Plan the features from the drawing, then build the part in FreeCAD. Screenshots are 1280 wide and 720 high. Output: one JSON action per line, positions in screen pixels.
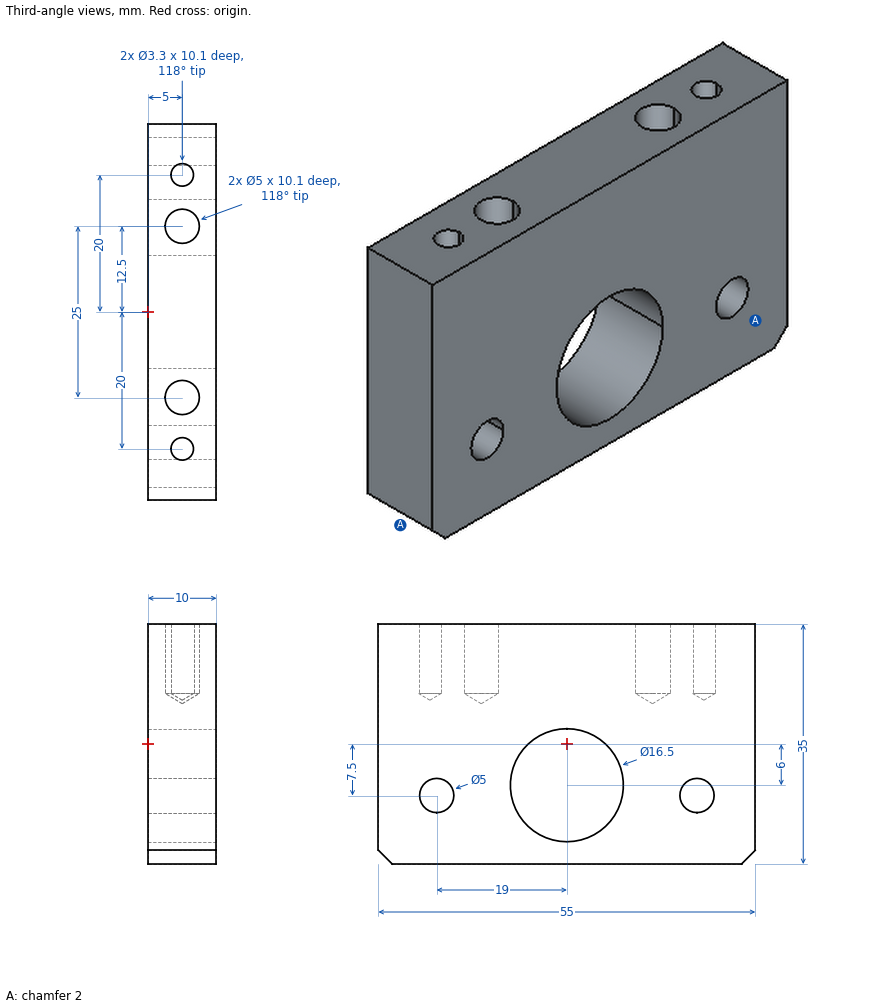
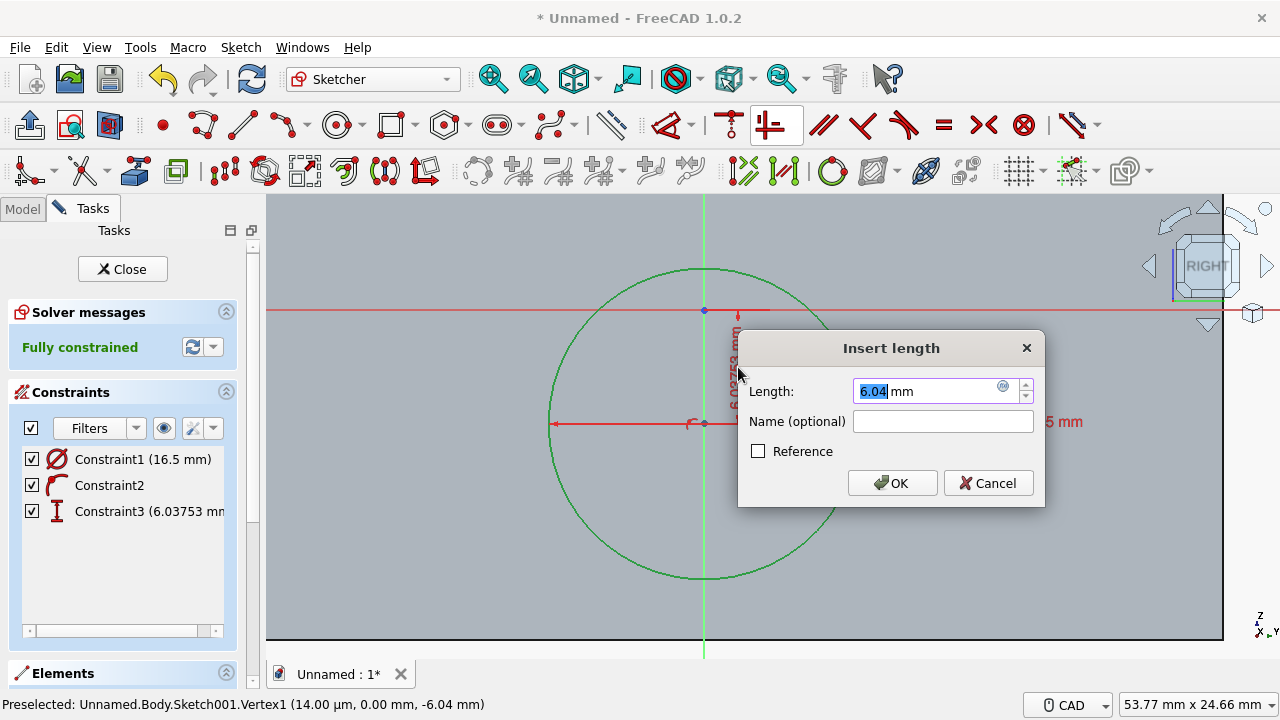
{"action": "type", "text": "6"}
{"action": "key", "text": "Return"}
{"action": "key", "text": "Escape"}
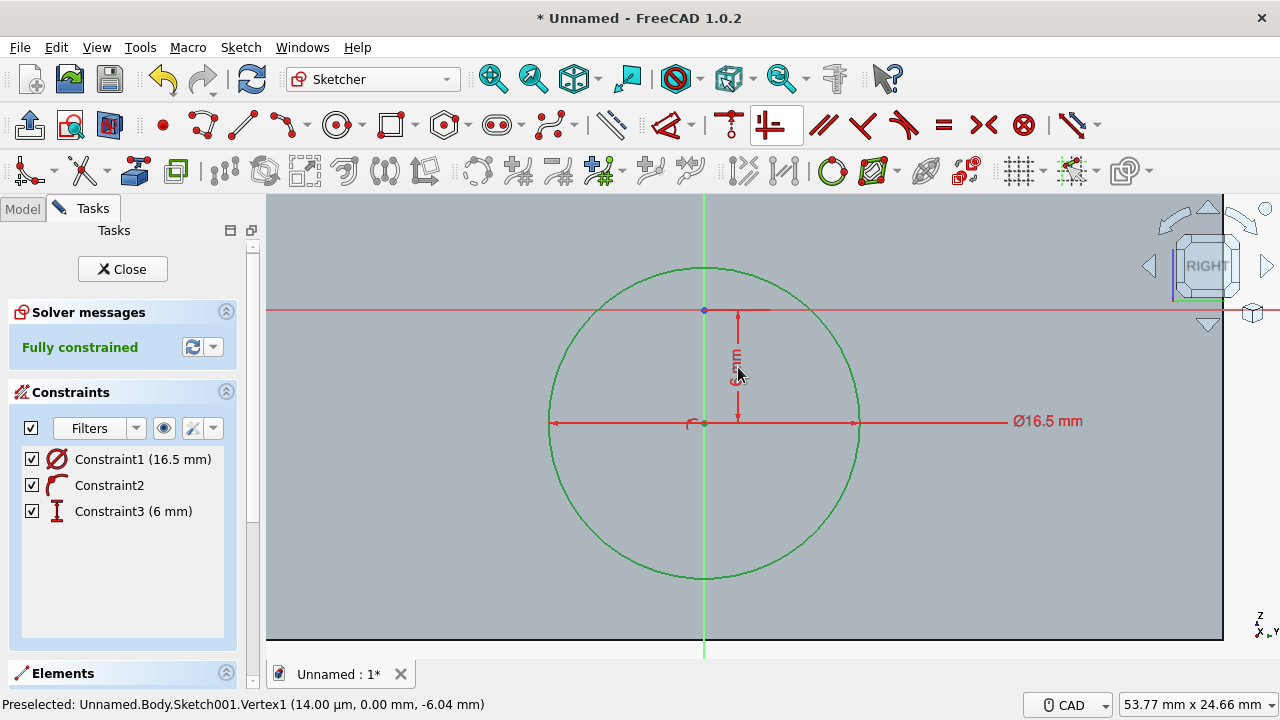
{"action": "left_click", "coordinate": [123, 269]}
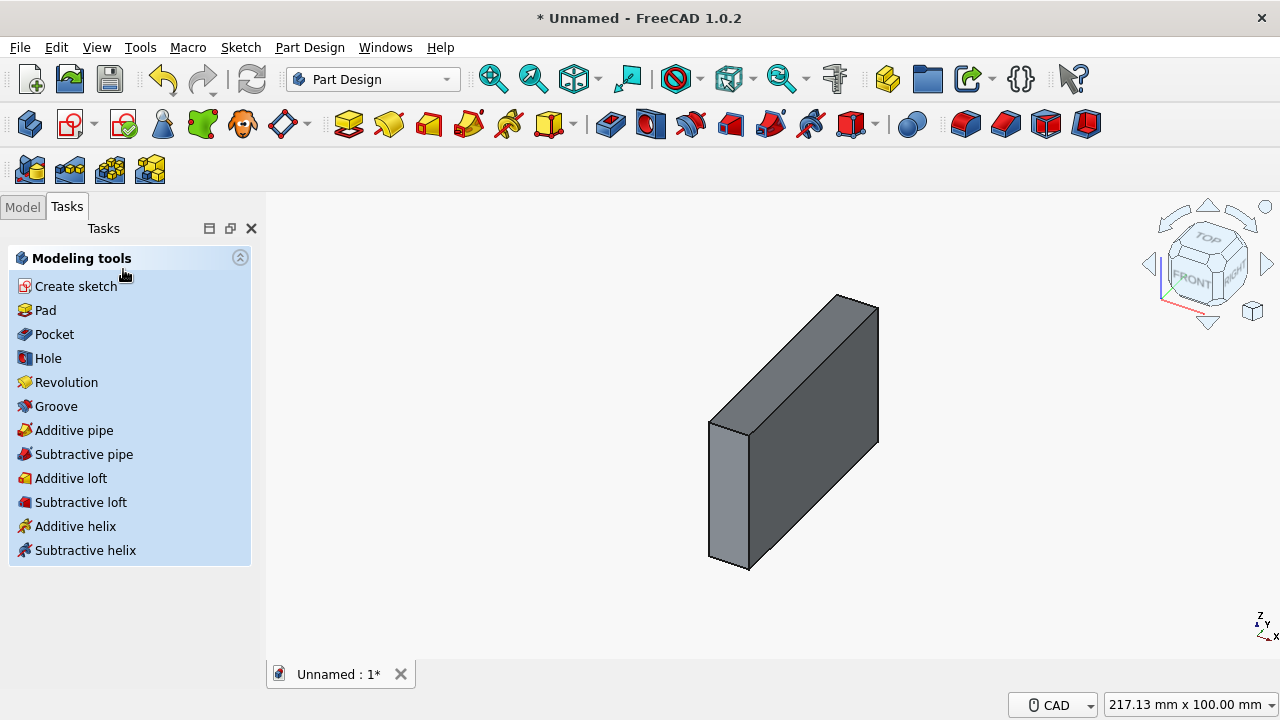
{"action": "left_click", "coordinate": [612, 124]}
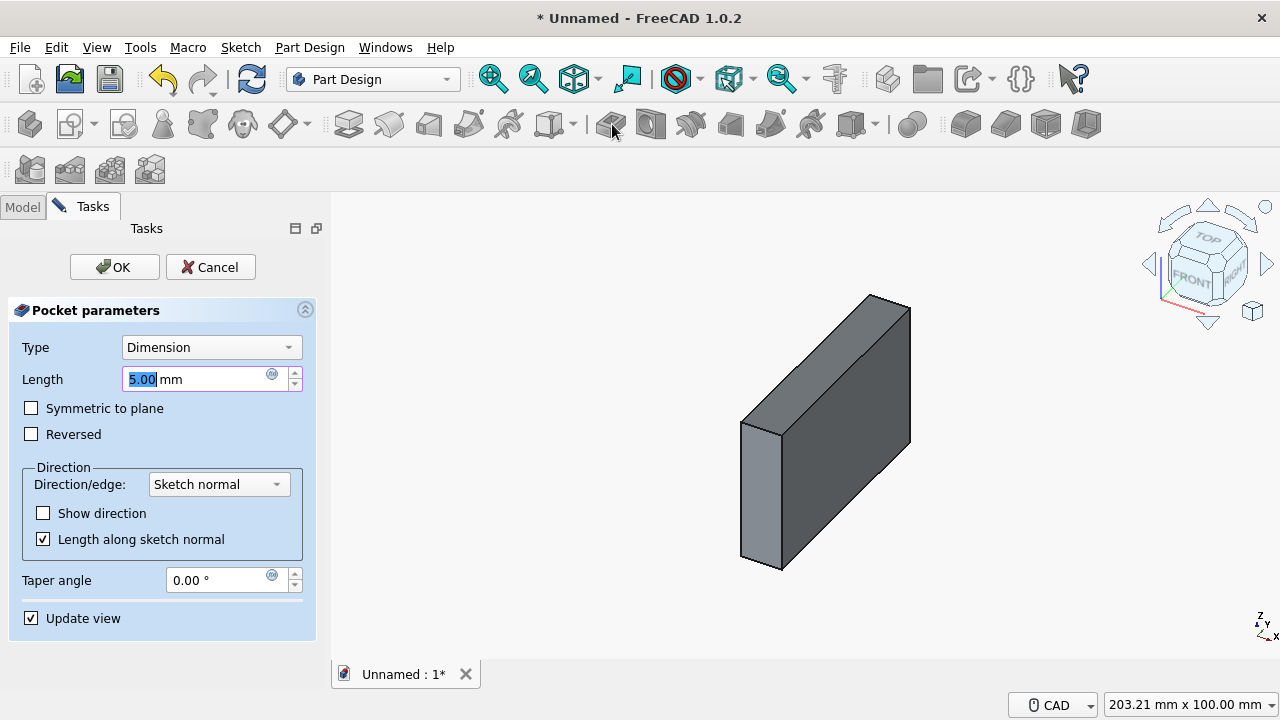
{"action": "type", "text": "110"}
{"action": "key", "text": "Tab"}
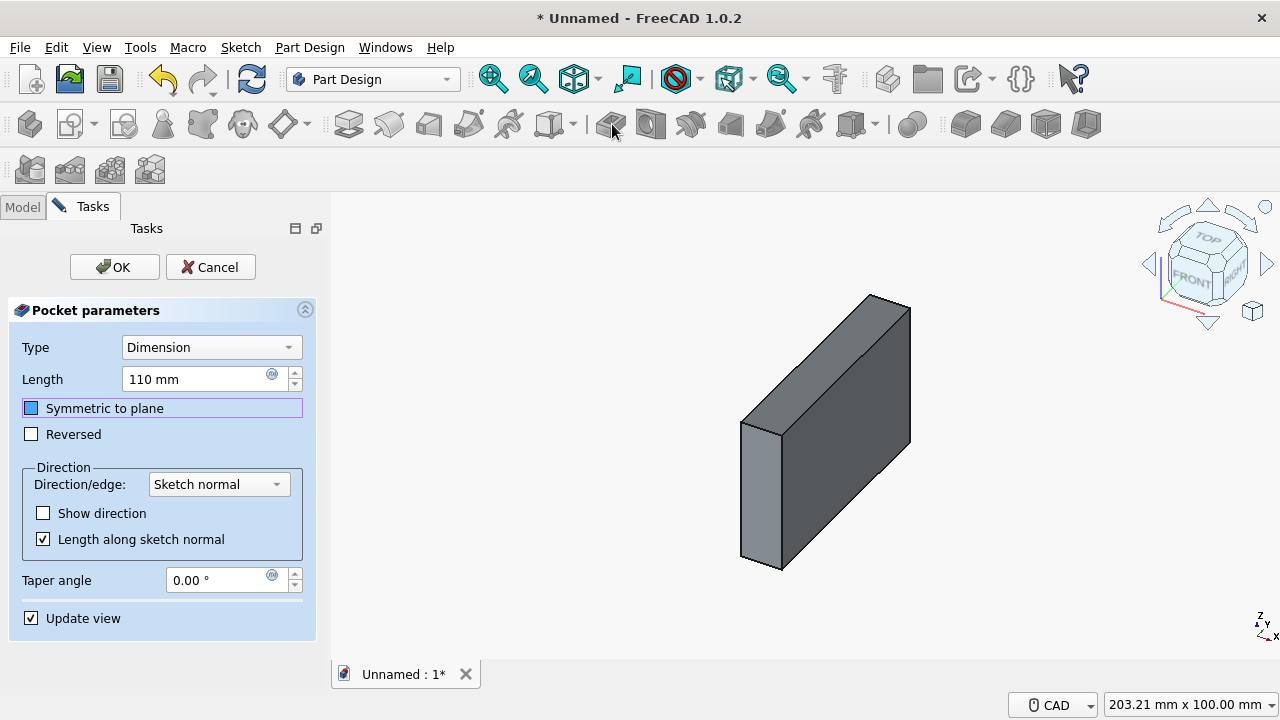
{"action": "left_click", "coordinate": [30, 434]}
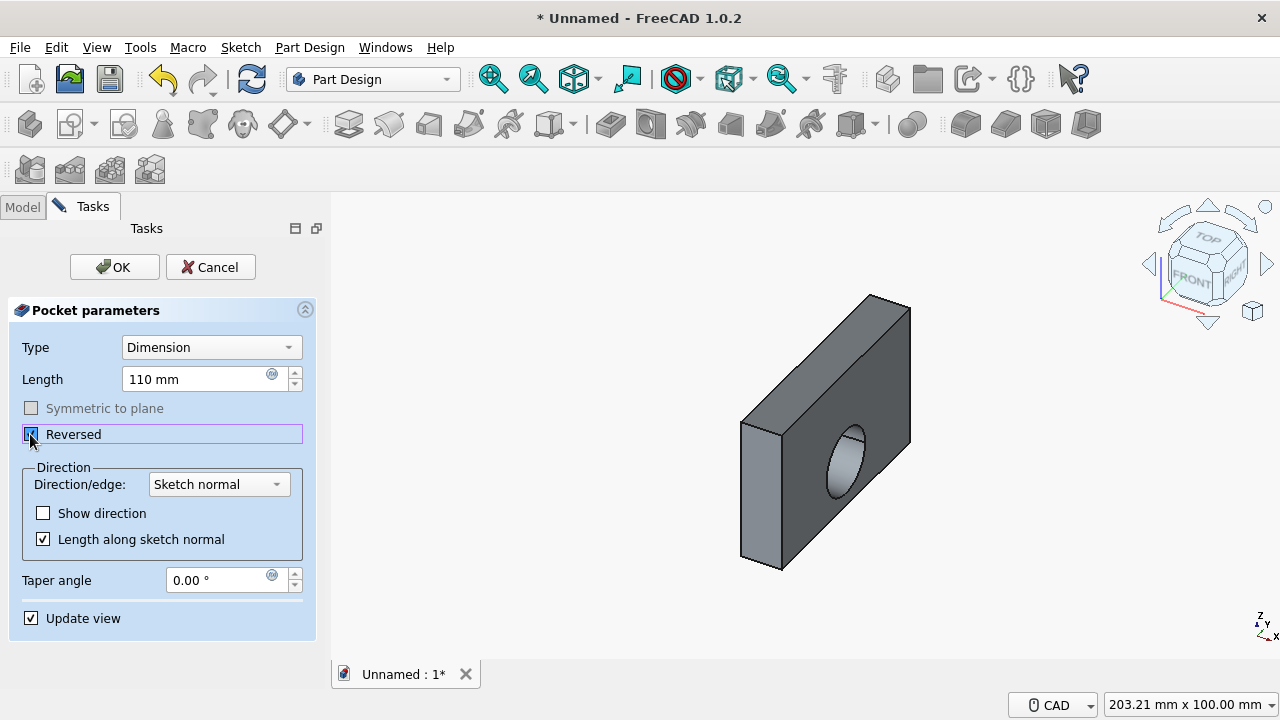
{"action": "left_click", "coordinate": [115, 267]}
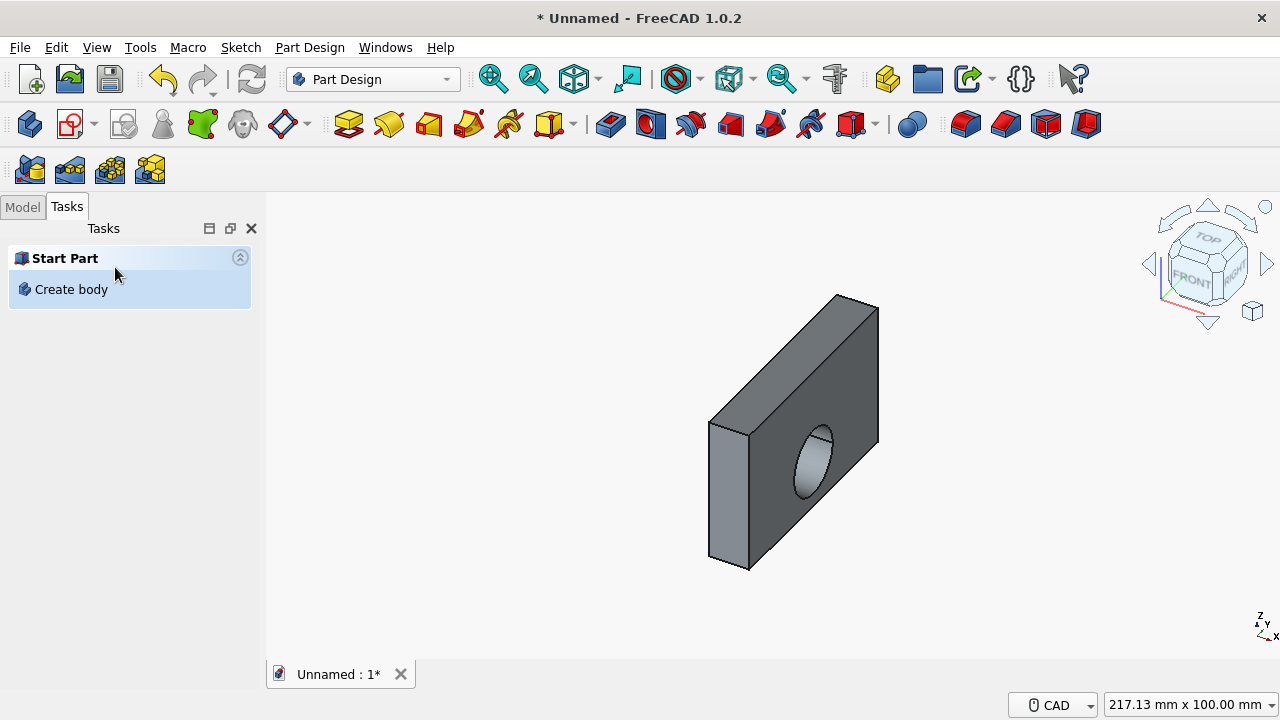
{"action": "left_click", "coordinate": [70, 124]}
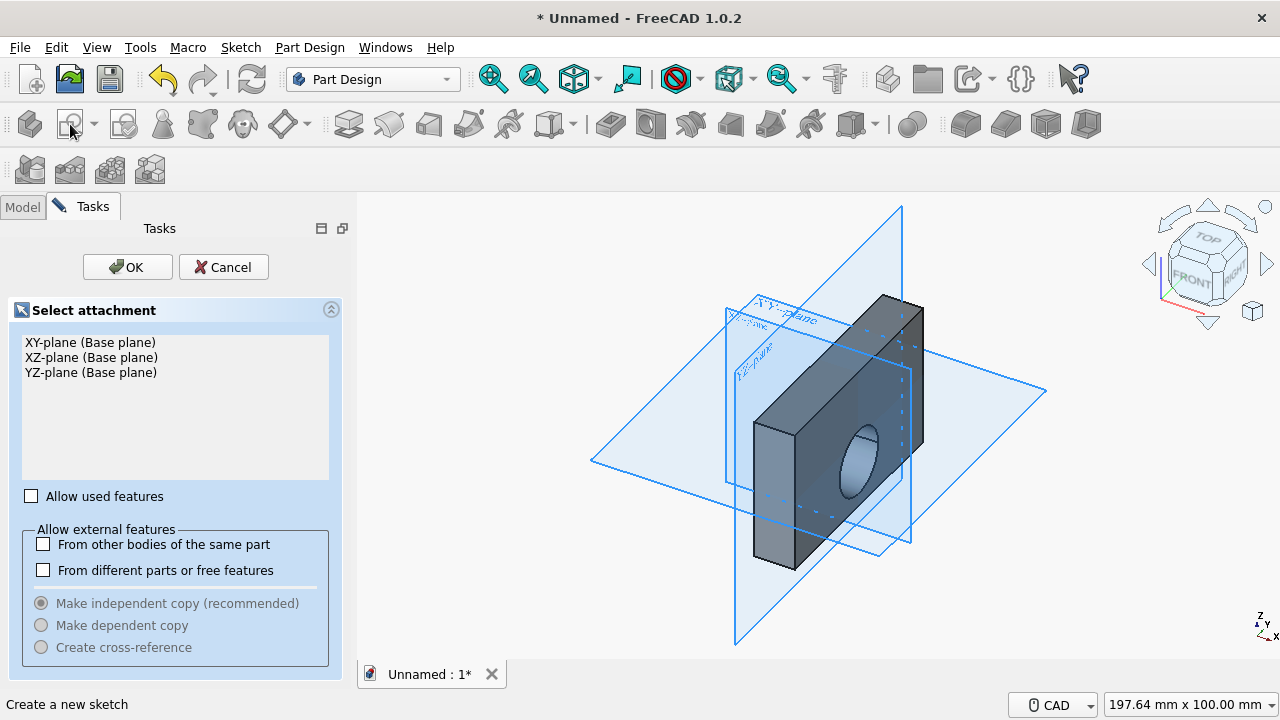
{"action": "left_click", "coordinate": [82, 372]}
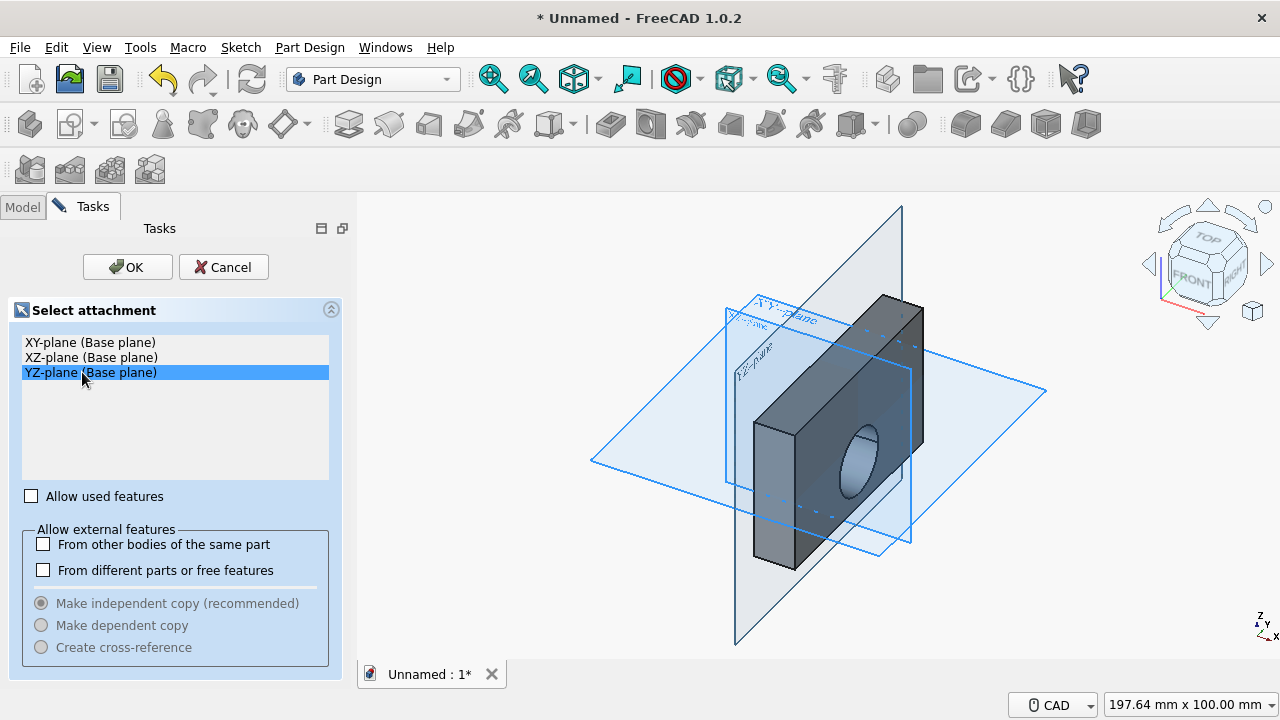
{"action": "left_click", "coordinate": [128, 267]}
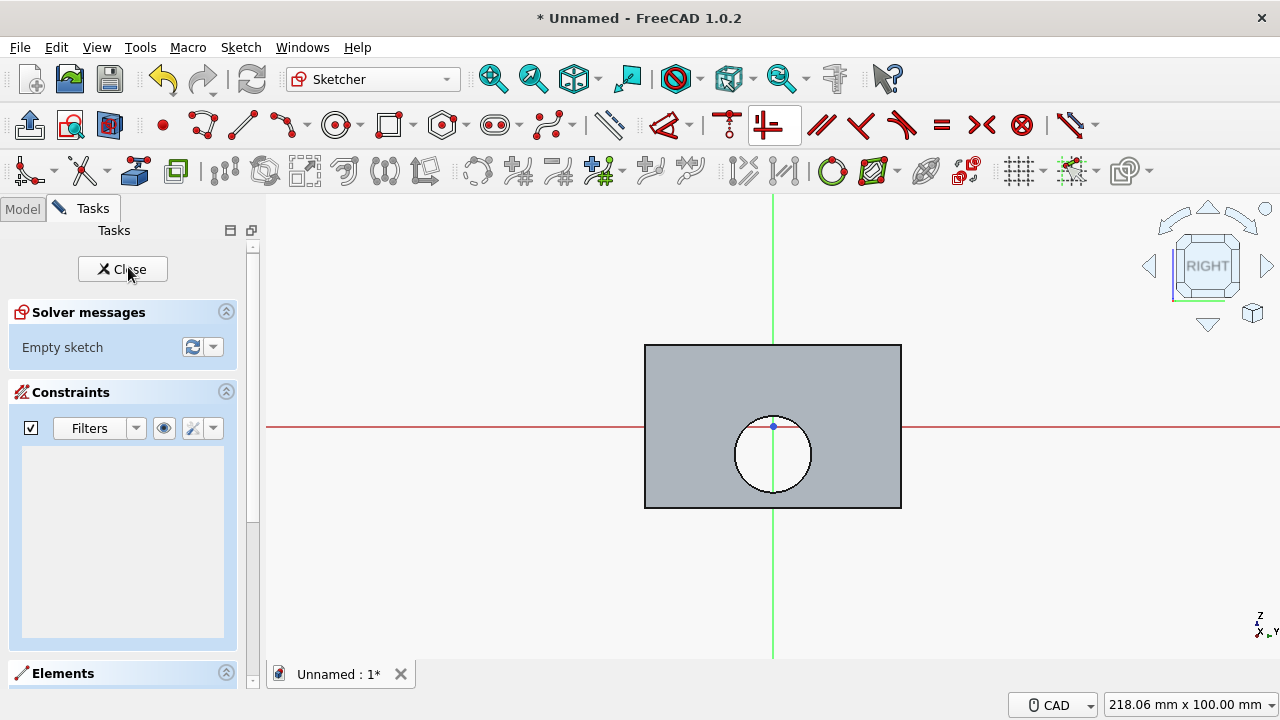
{"action": "left_click", "coordinate": [110, 126]}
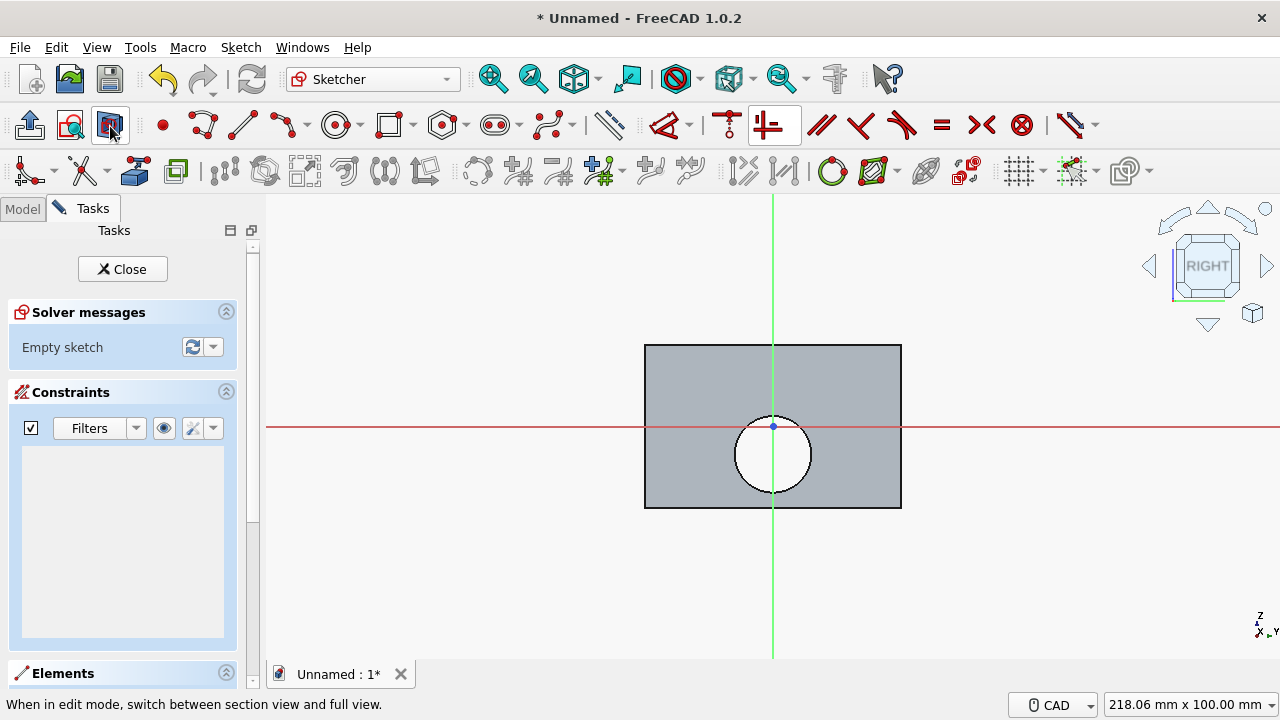
{"action": "scroll", "coordinate": [683, 464], "scroll_direction": "up", "scroll_amount": 13}